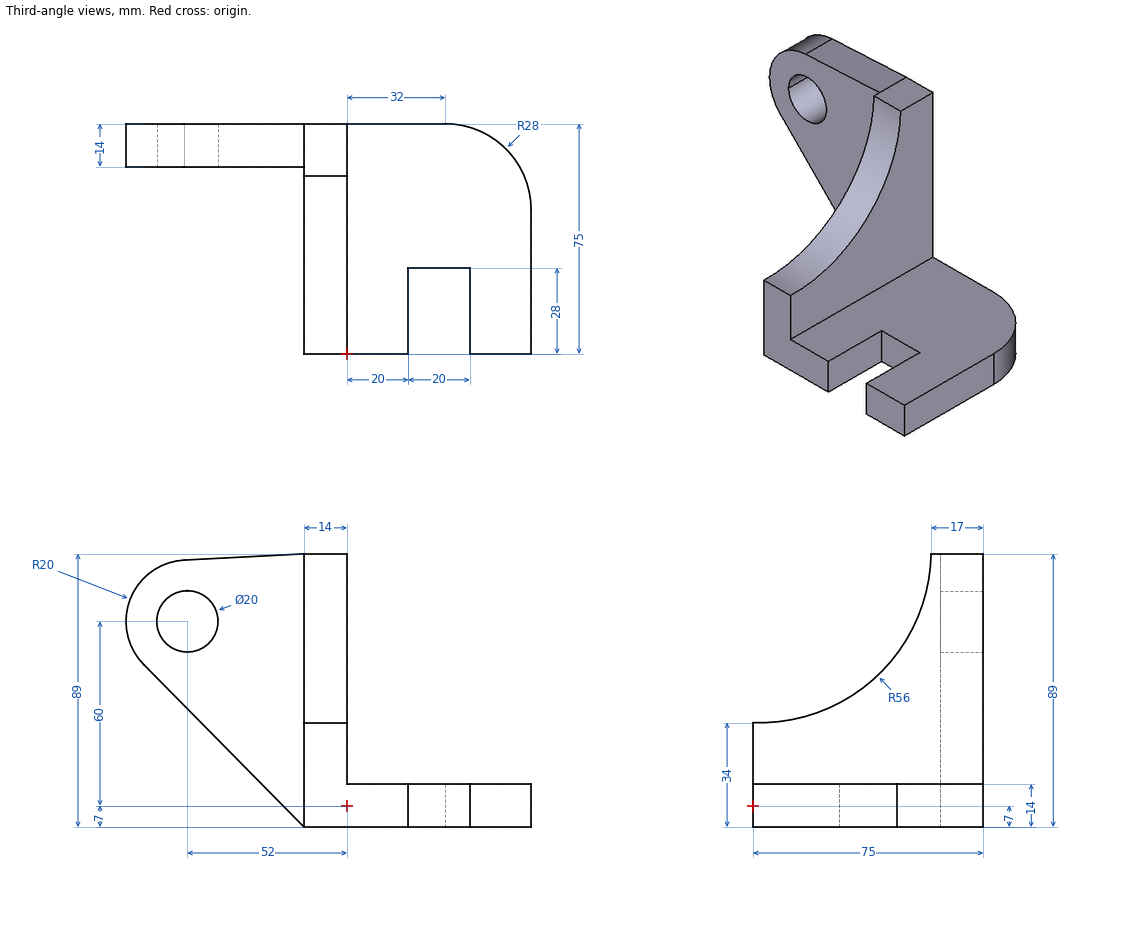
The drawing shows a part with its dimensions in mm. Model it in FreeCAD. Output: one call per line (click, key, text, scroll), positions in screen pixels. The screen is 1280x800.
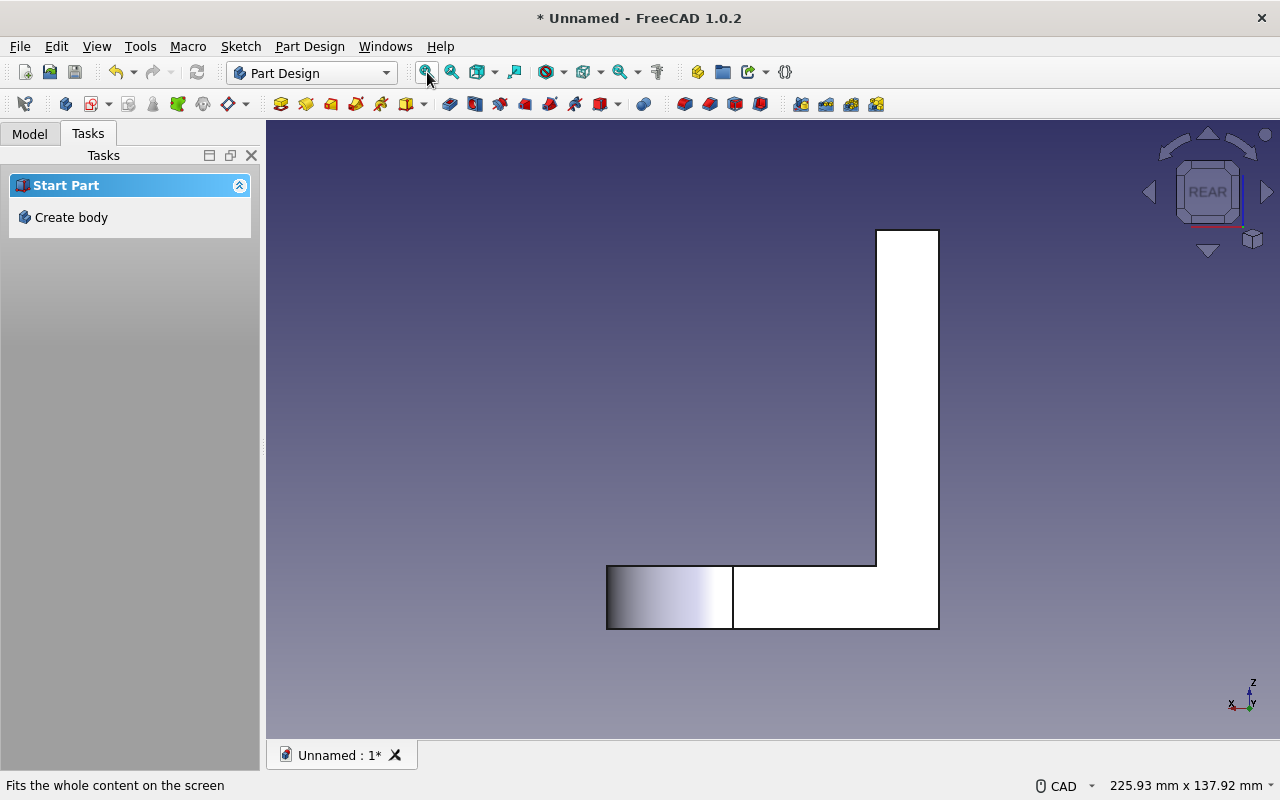
click(777, 600)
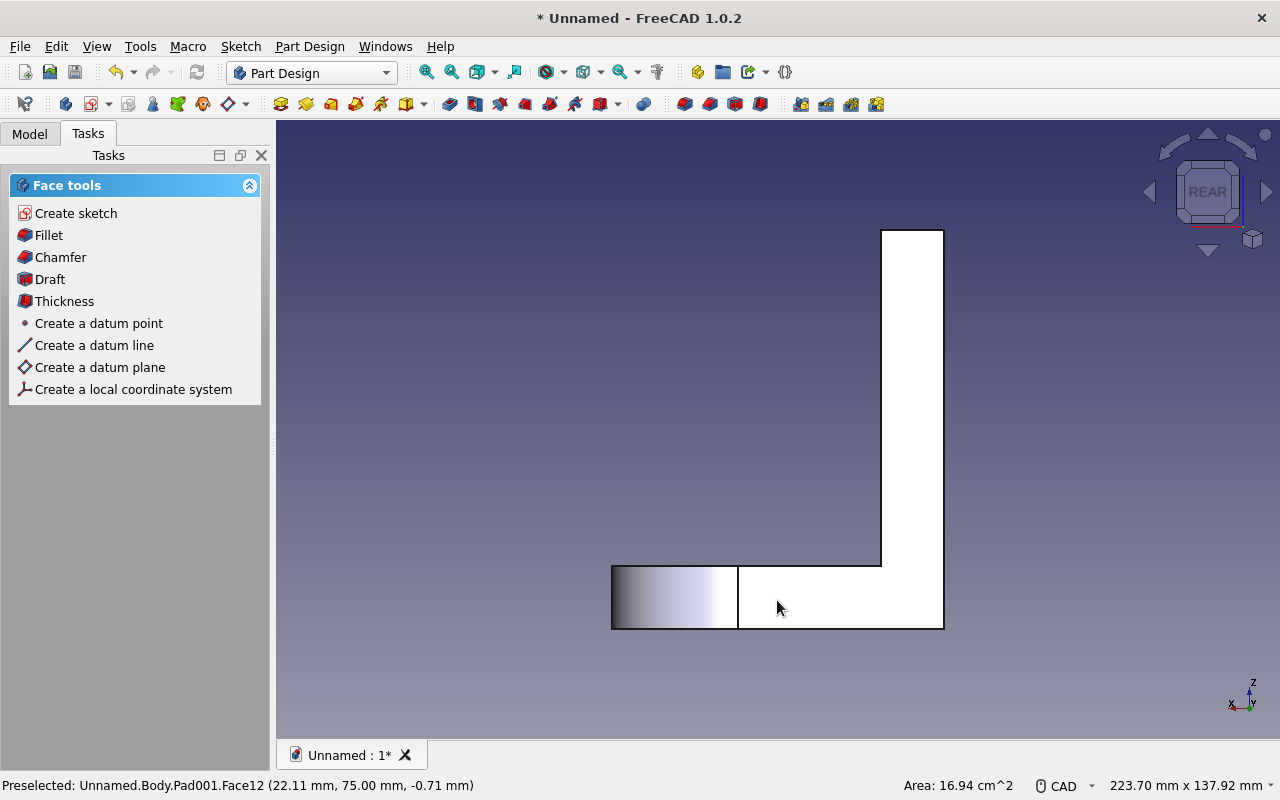
click(90, 104)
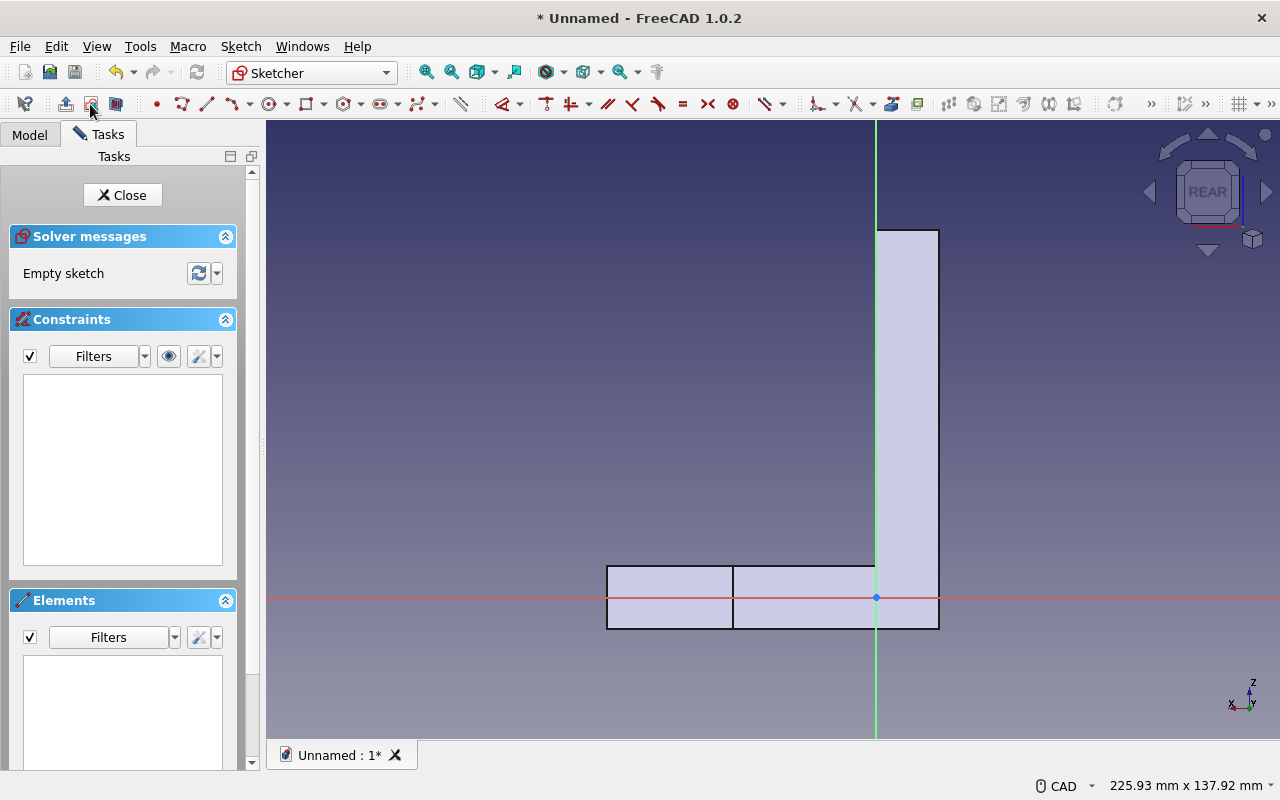
scroll(294, 430, down, 1)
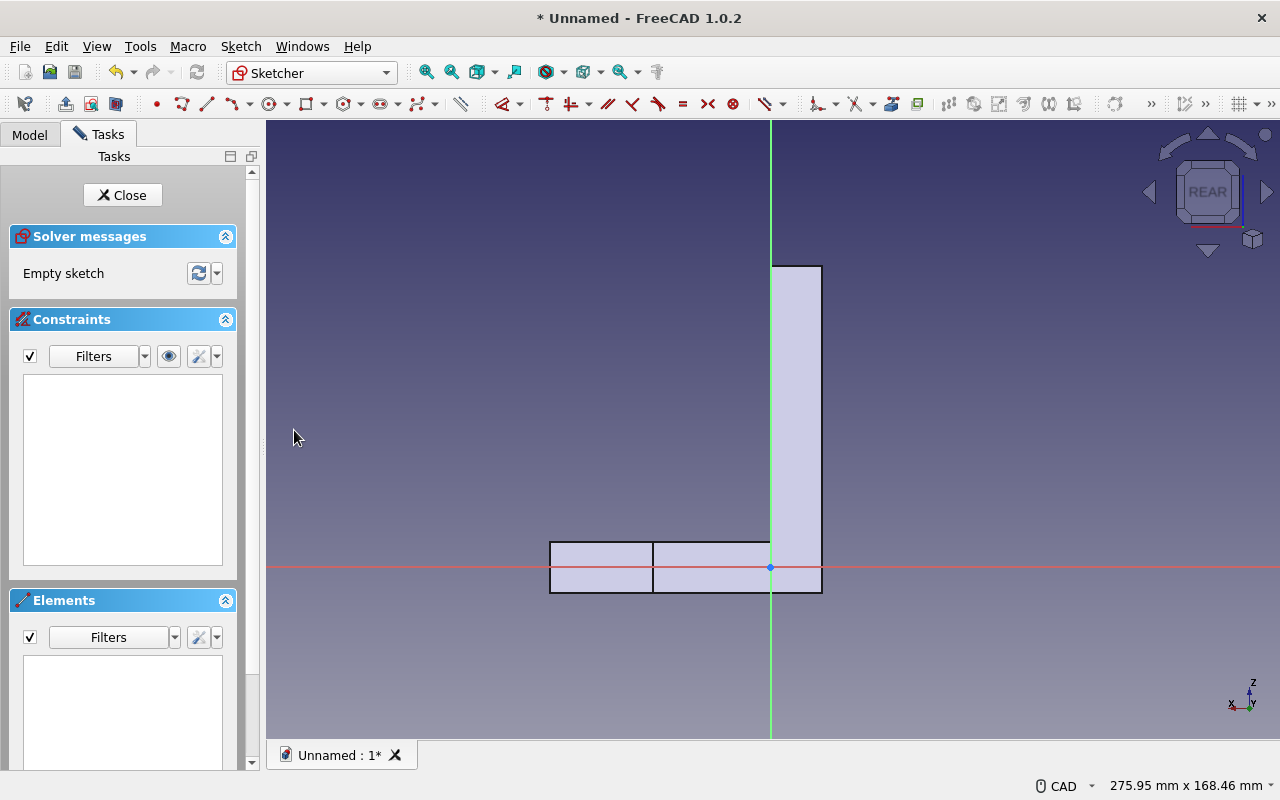
click(182, 104)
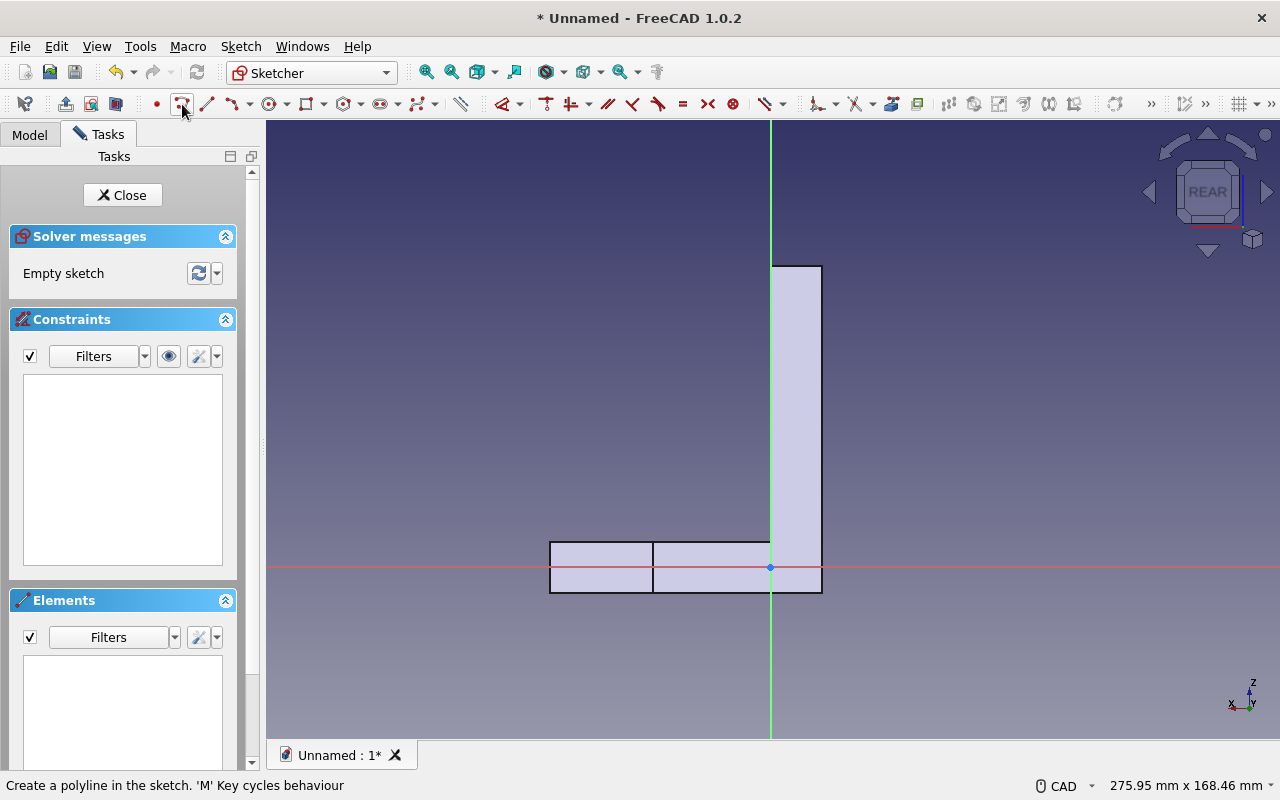
click(966, 274)
click(822, 266)
click(822, 593)
click(1014, 399)
right_click(1014, 399)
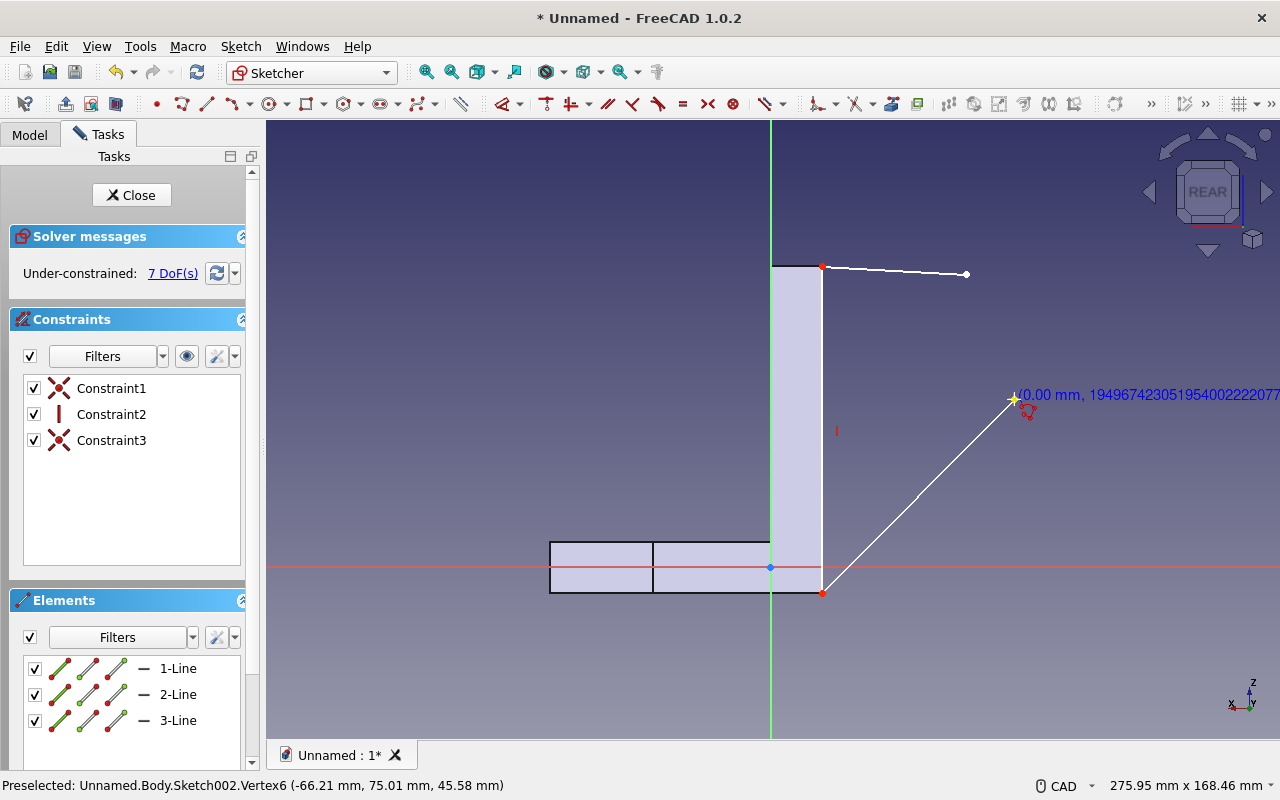
click(232, 104)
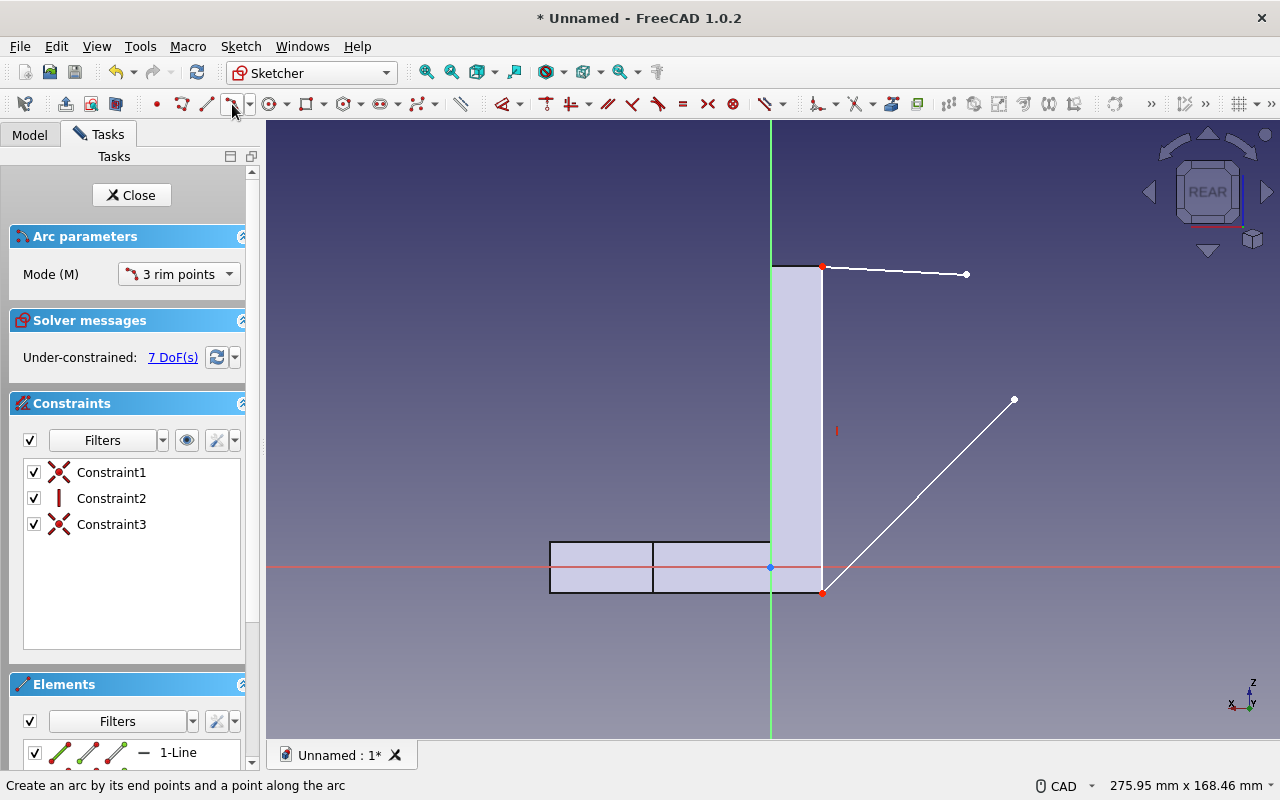
click(1014, 400)
click(966, 275)
click(1030, 320)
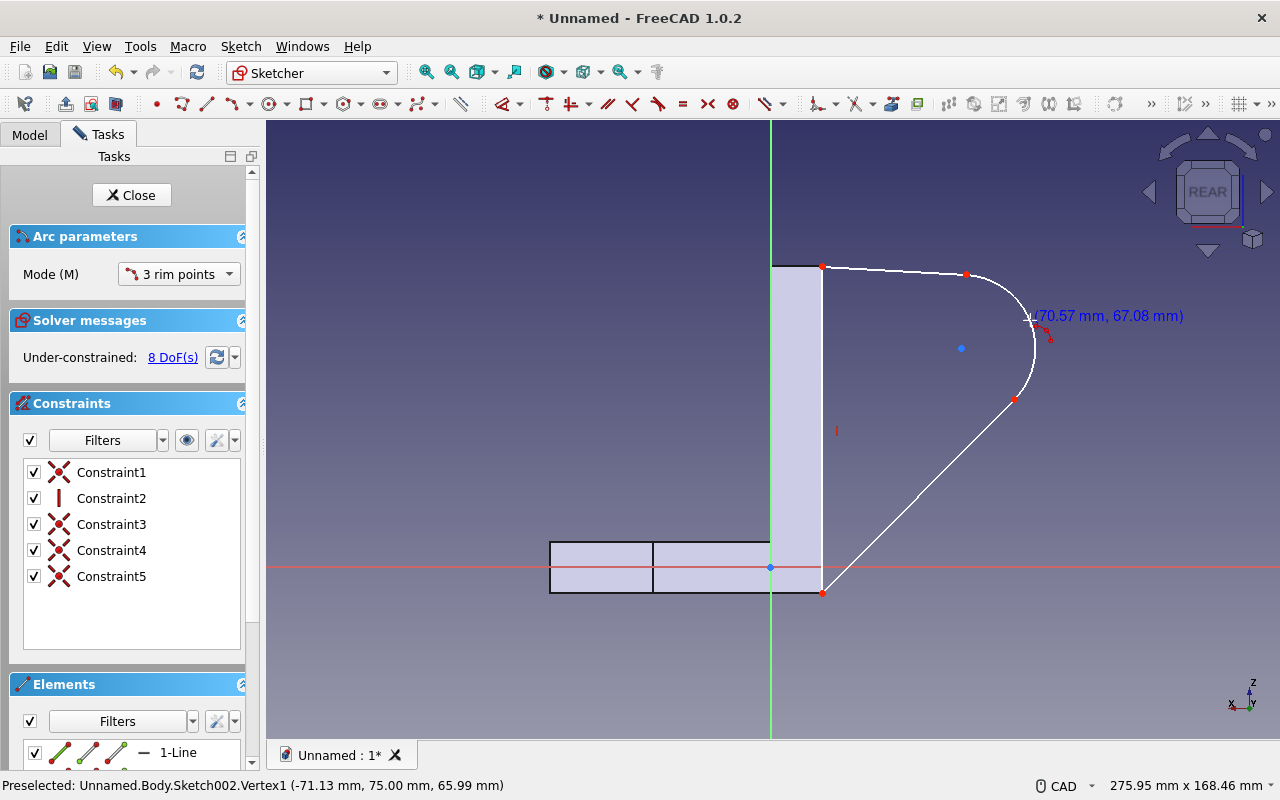
click(268, 104)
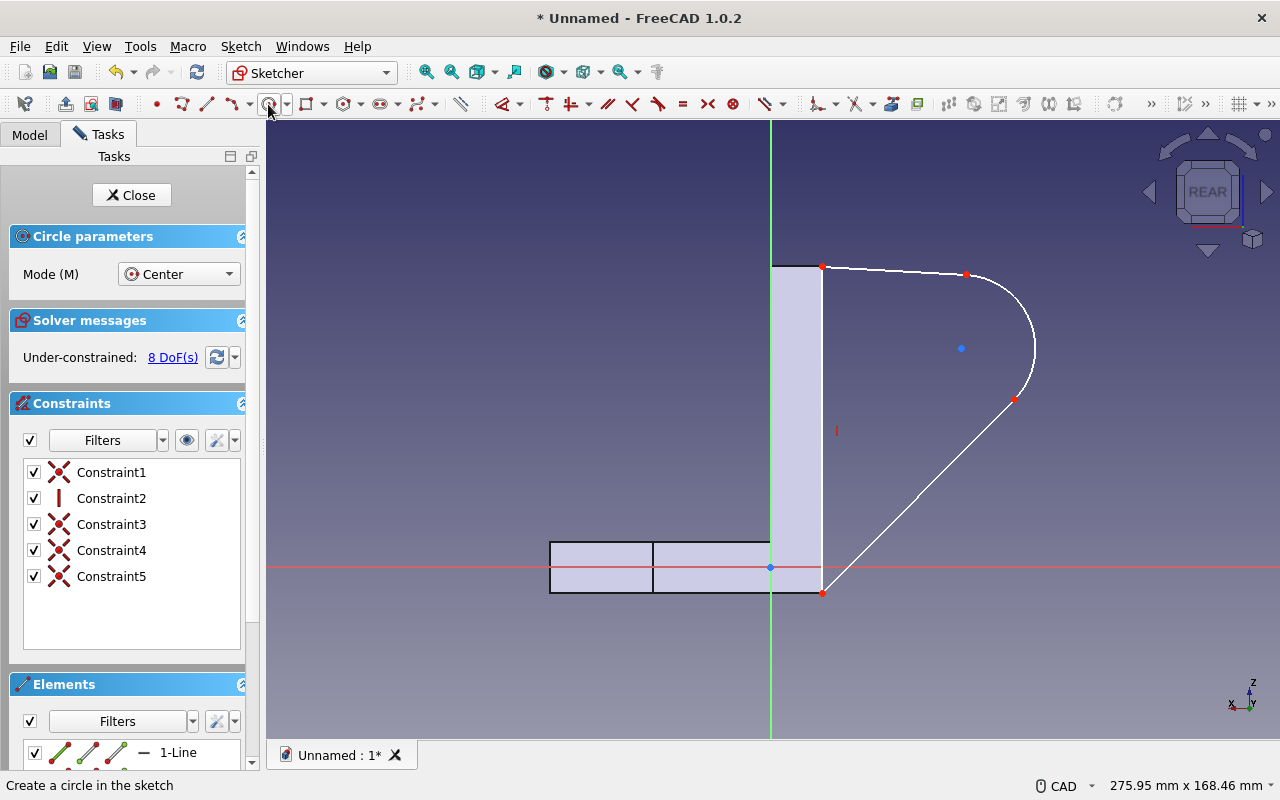
click(962, 347)
click(988, 321)
key(Escape)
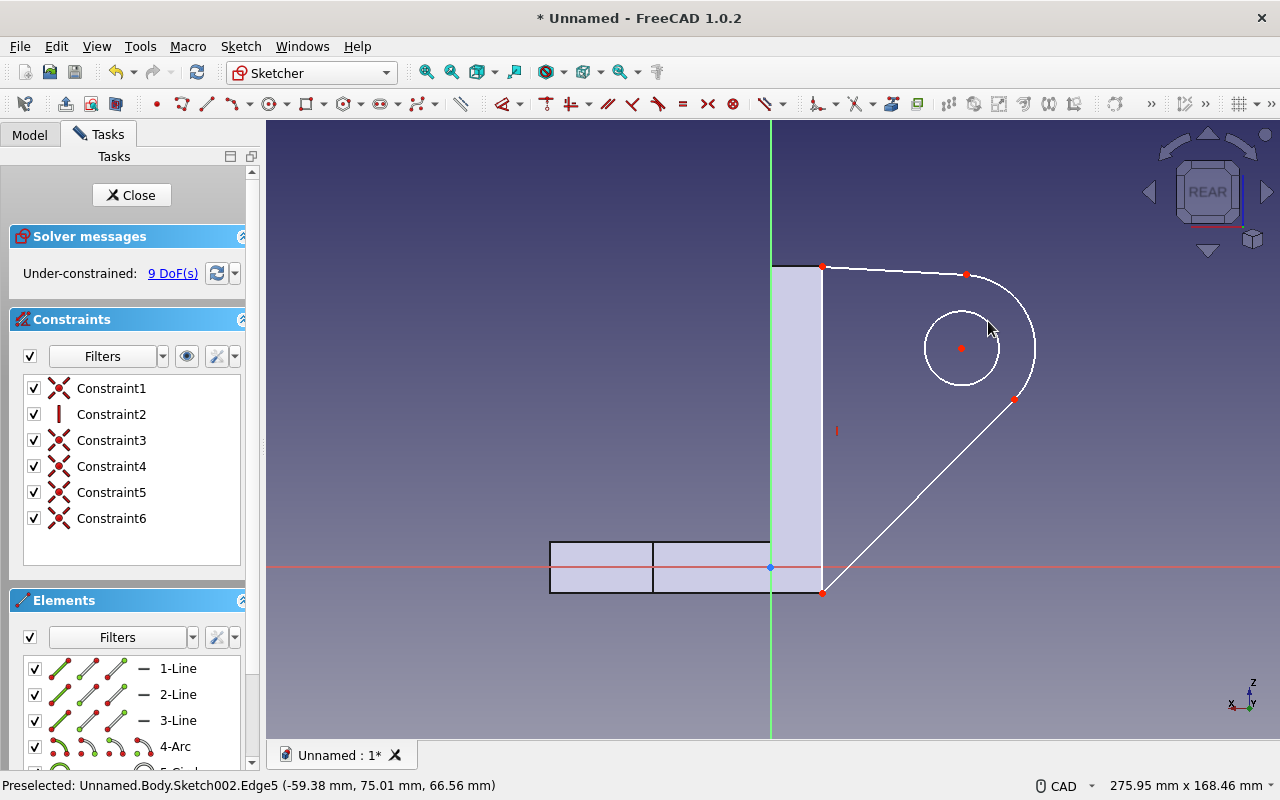
click(923, 273)